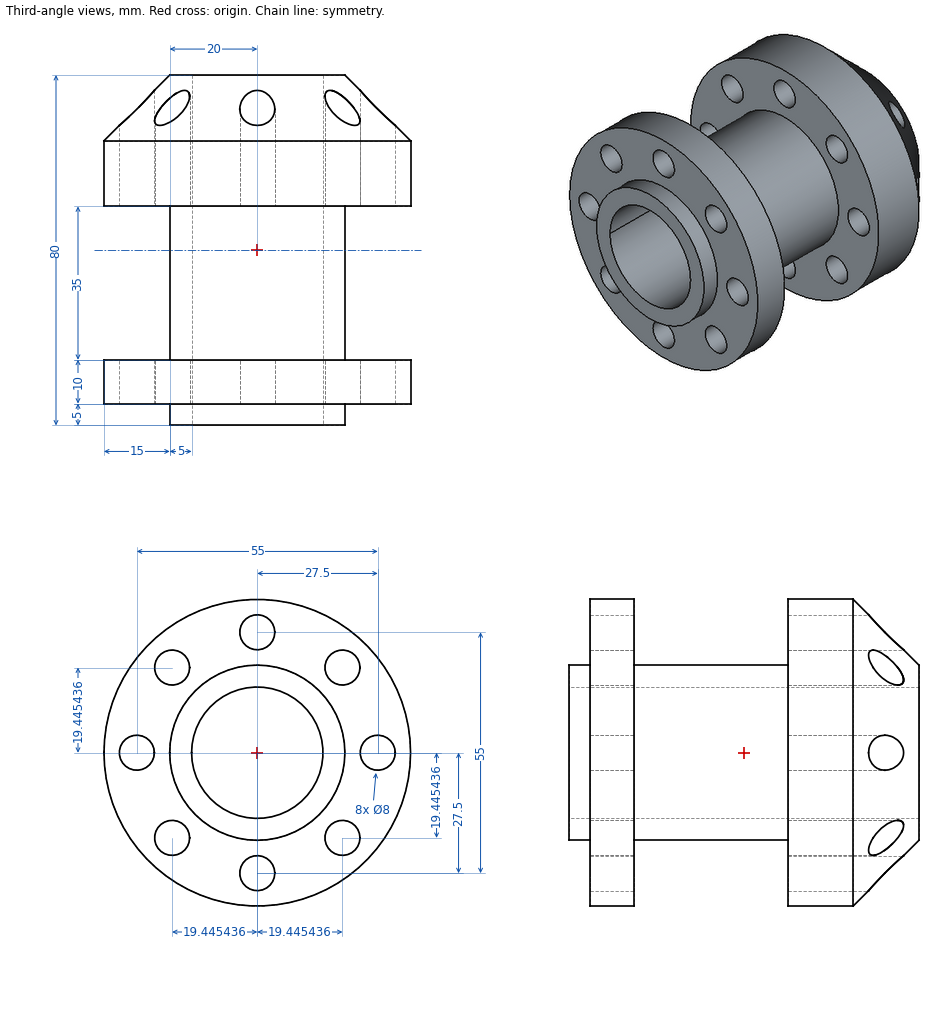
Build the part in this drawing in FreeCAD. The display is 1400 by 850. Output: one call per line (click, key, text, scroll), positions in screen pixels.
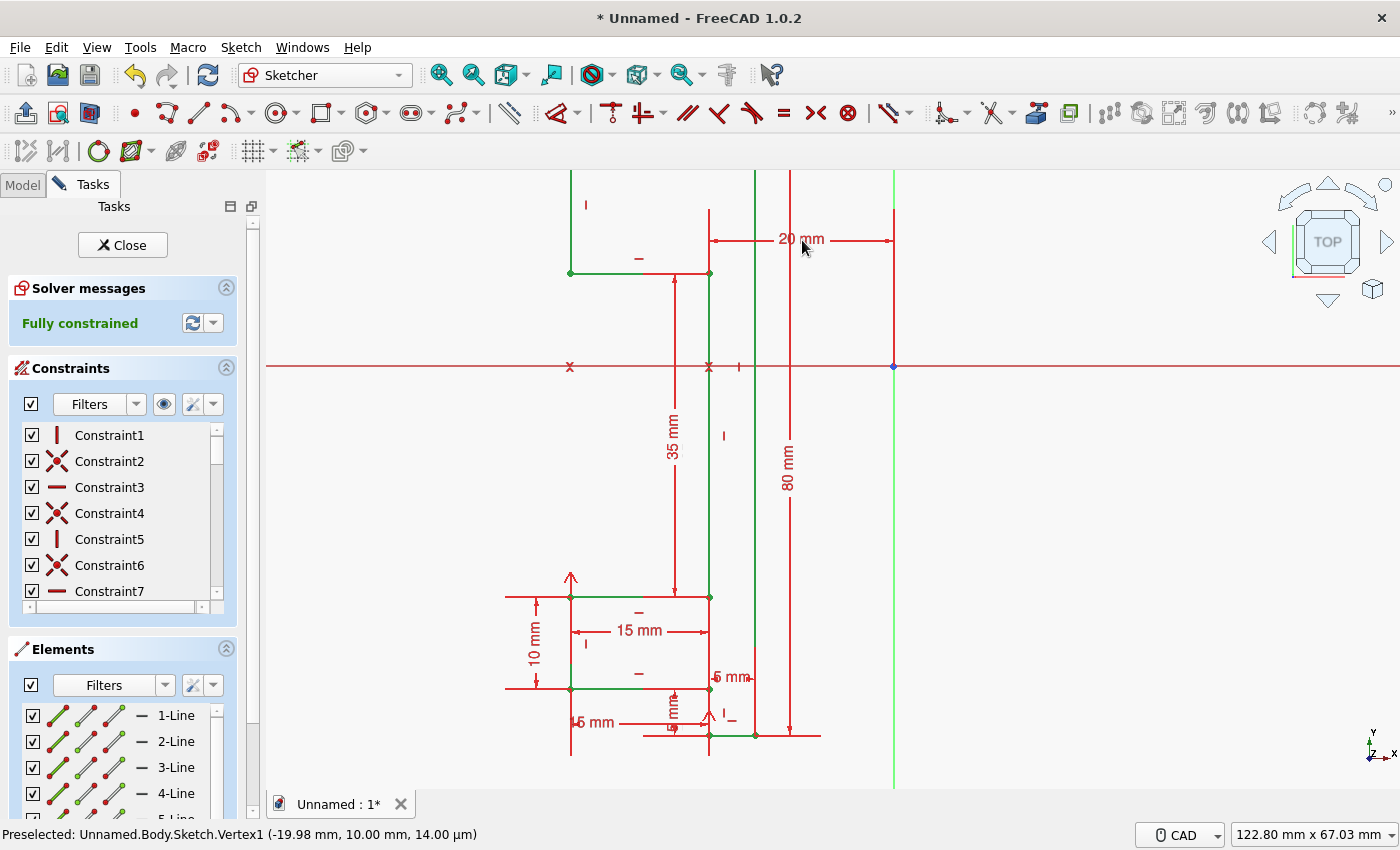
click(123, 245)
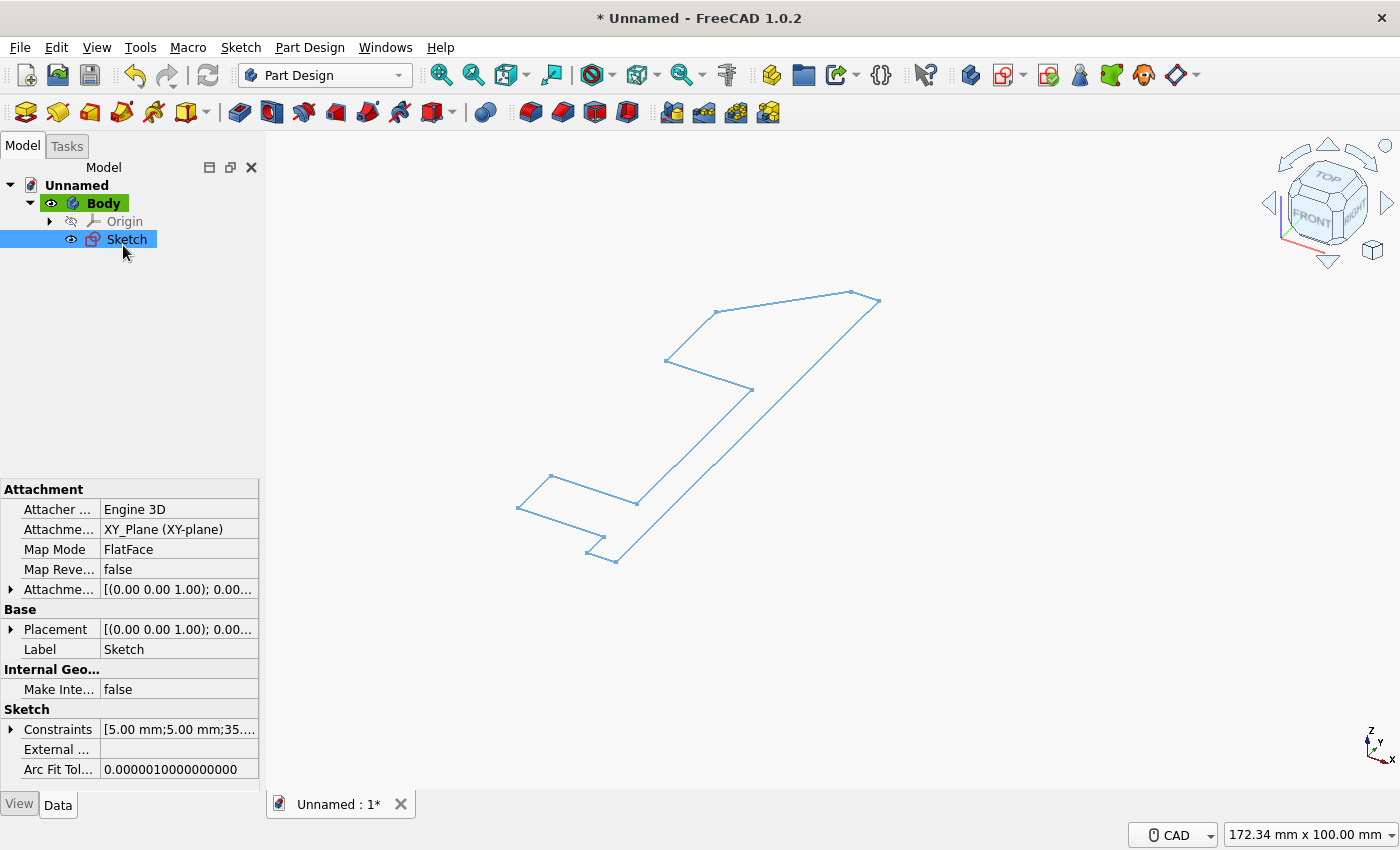
click(58, 112)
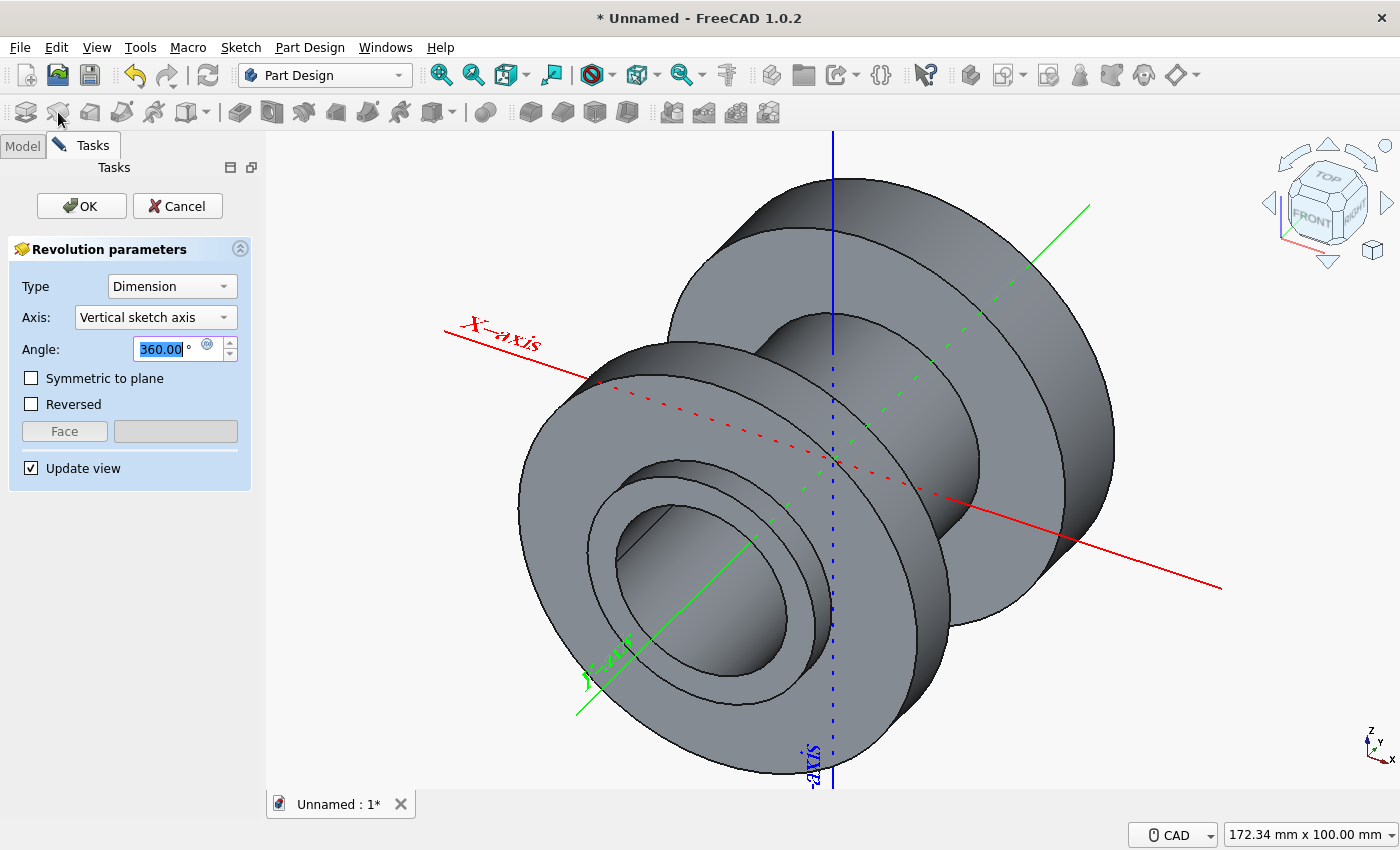
click(82, 206)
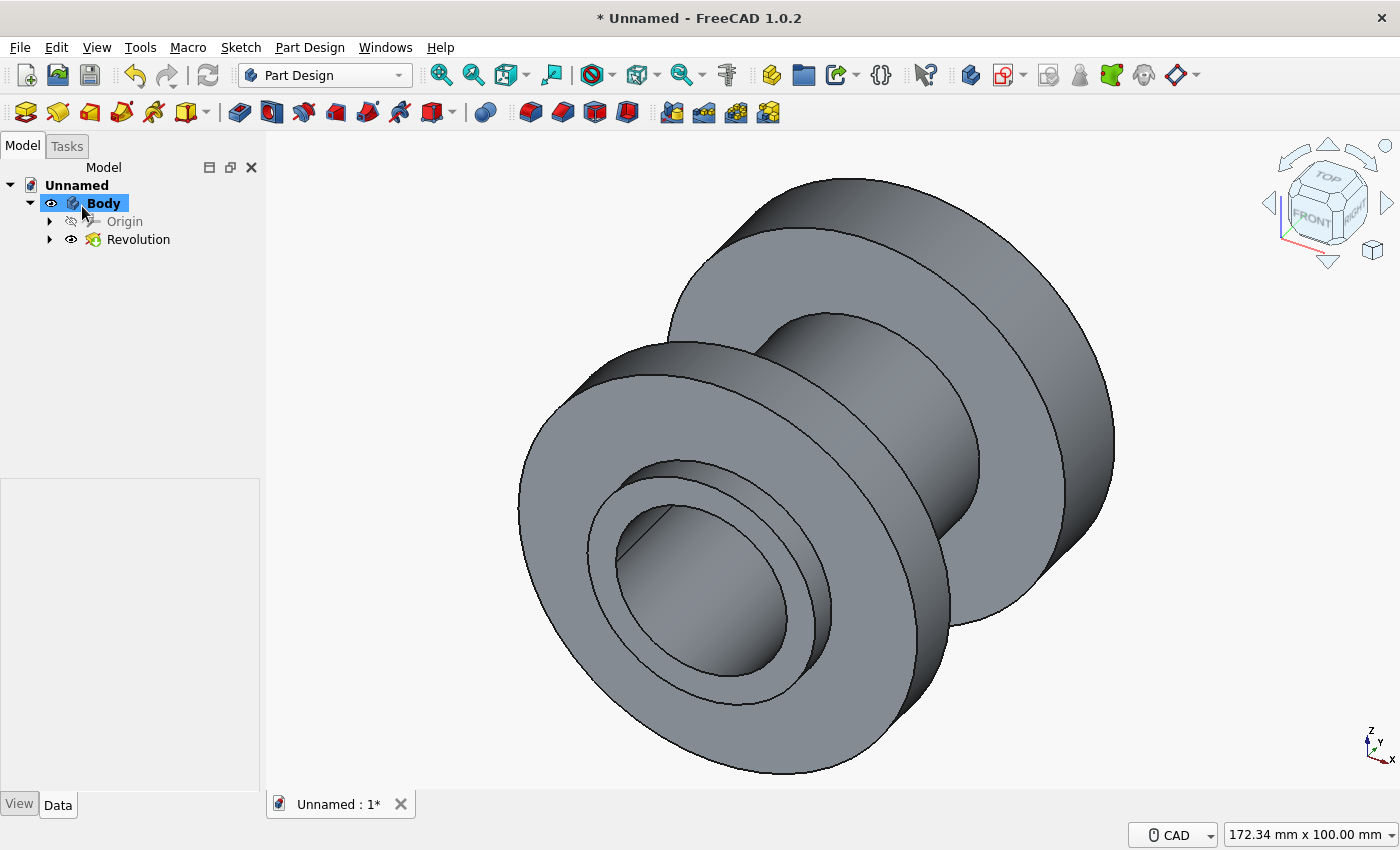
key(v)
key(f)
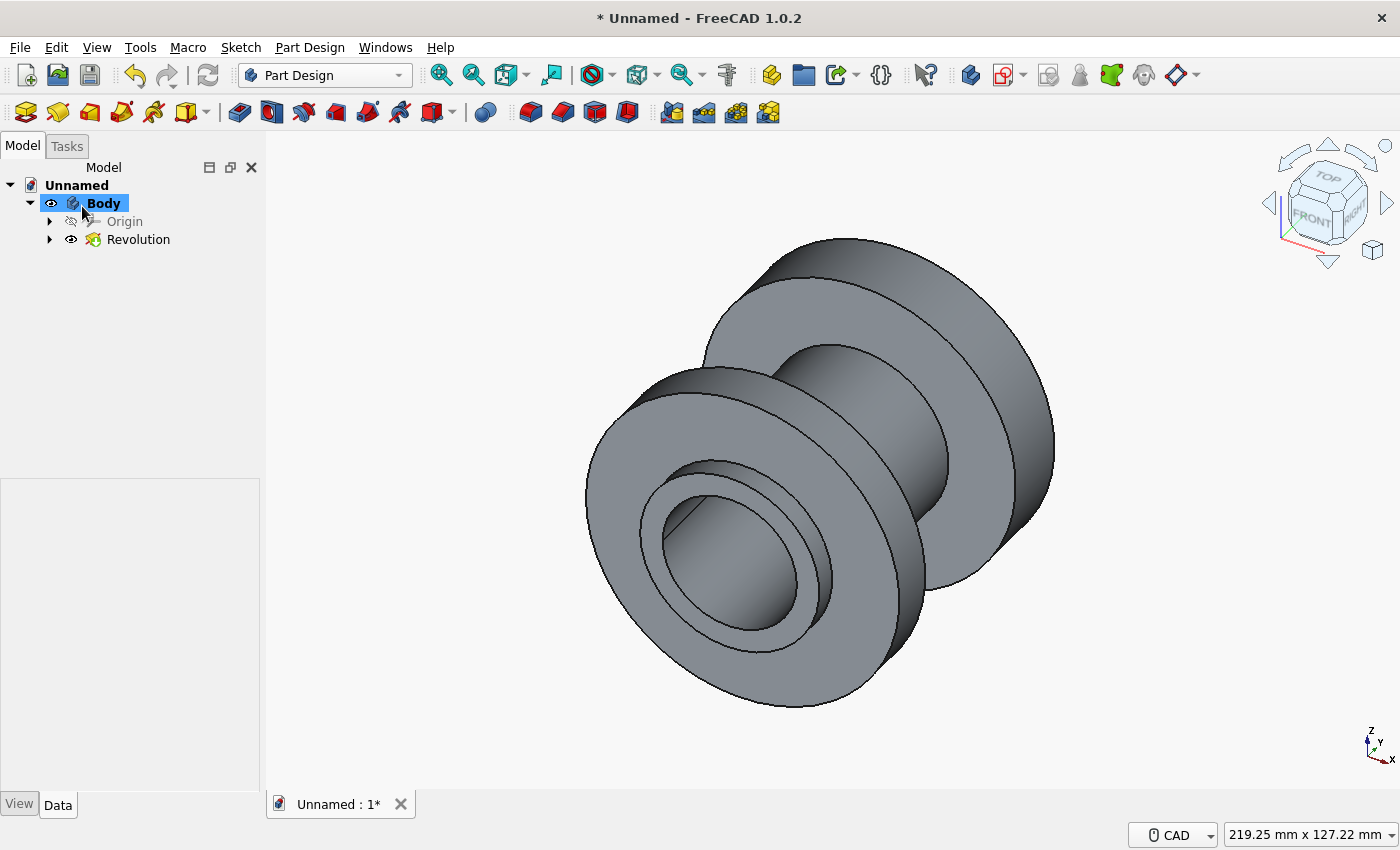
click(832, 663)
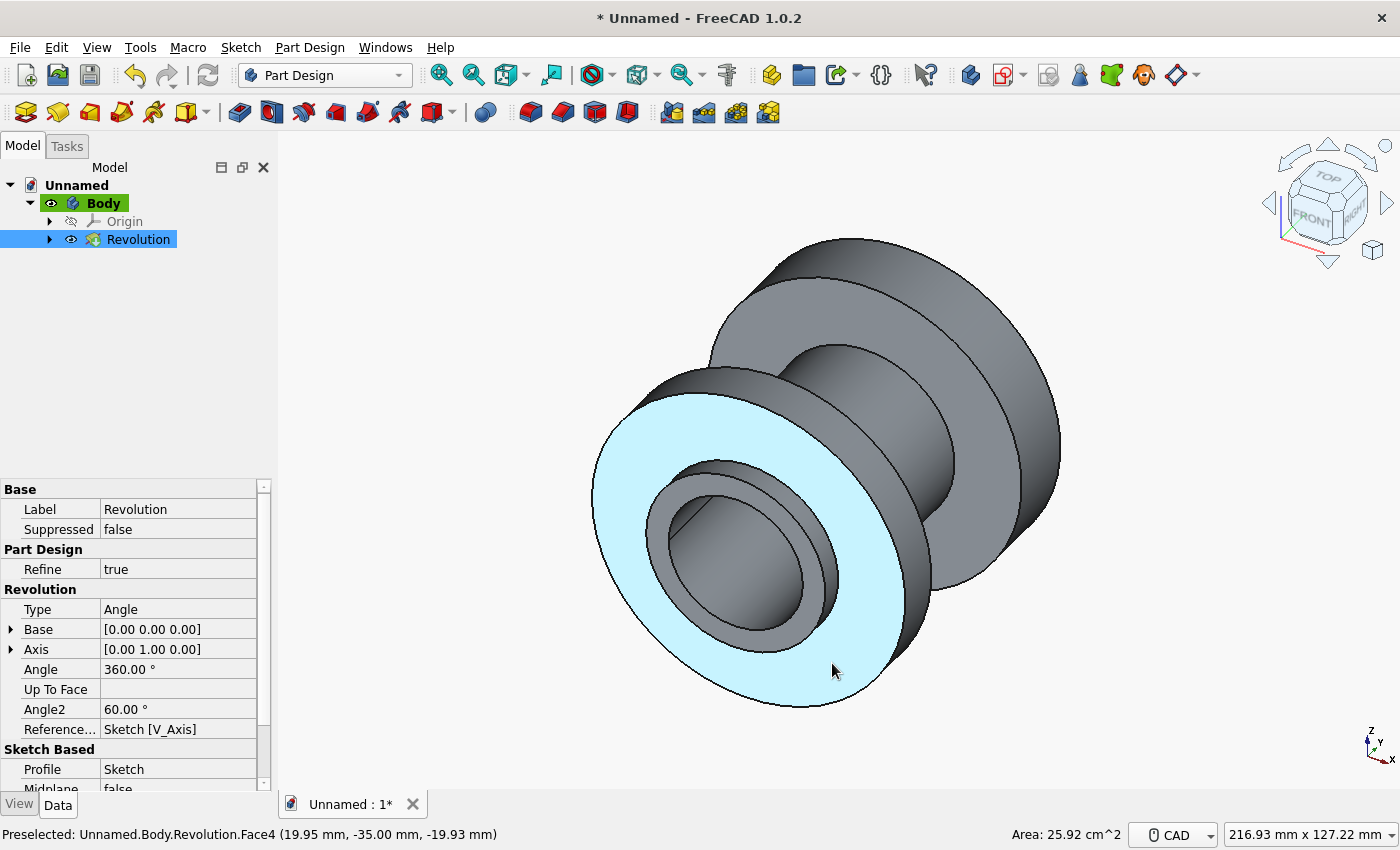
click(1004, 76)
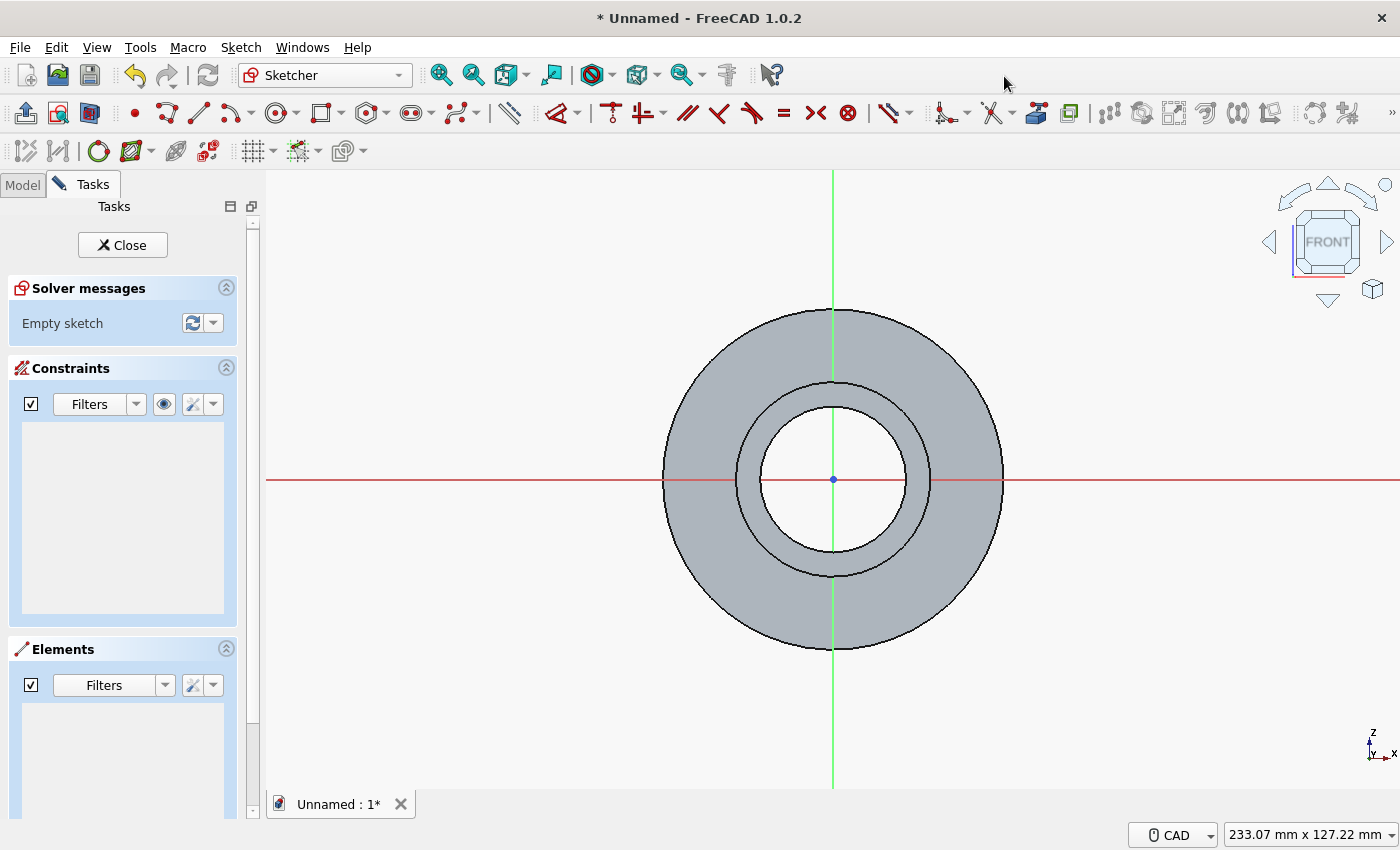
key(g)
key(c)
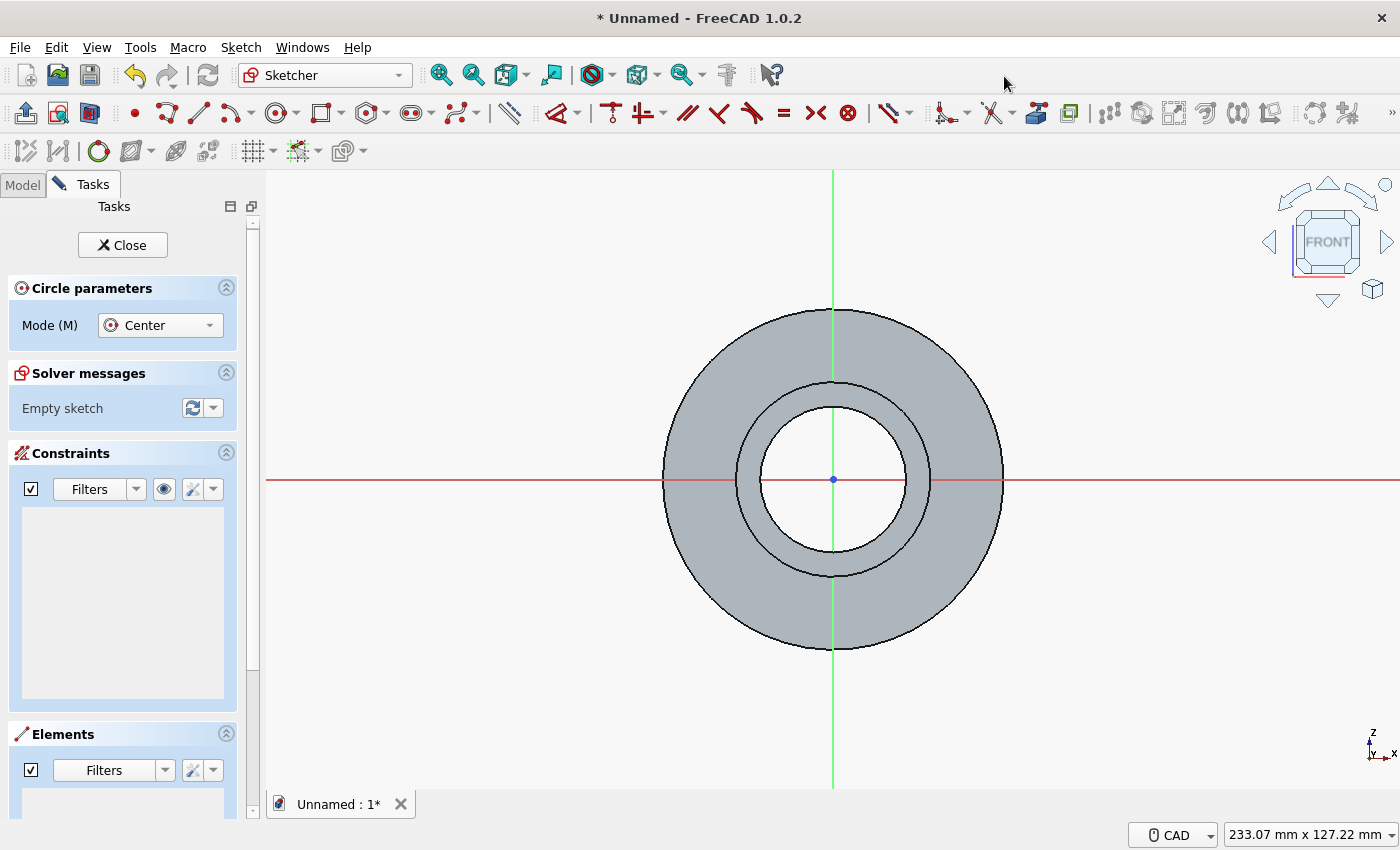
click(967, 480)
click(974, 461)